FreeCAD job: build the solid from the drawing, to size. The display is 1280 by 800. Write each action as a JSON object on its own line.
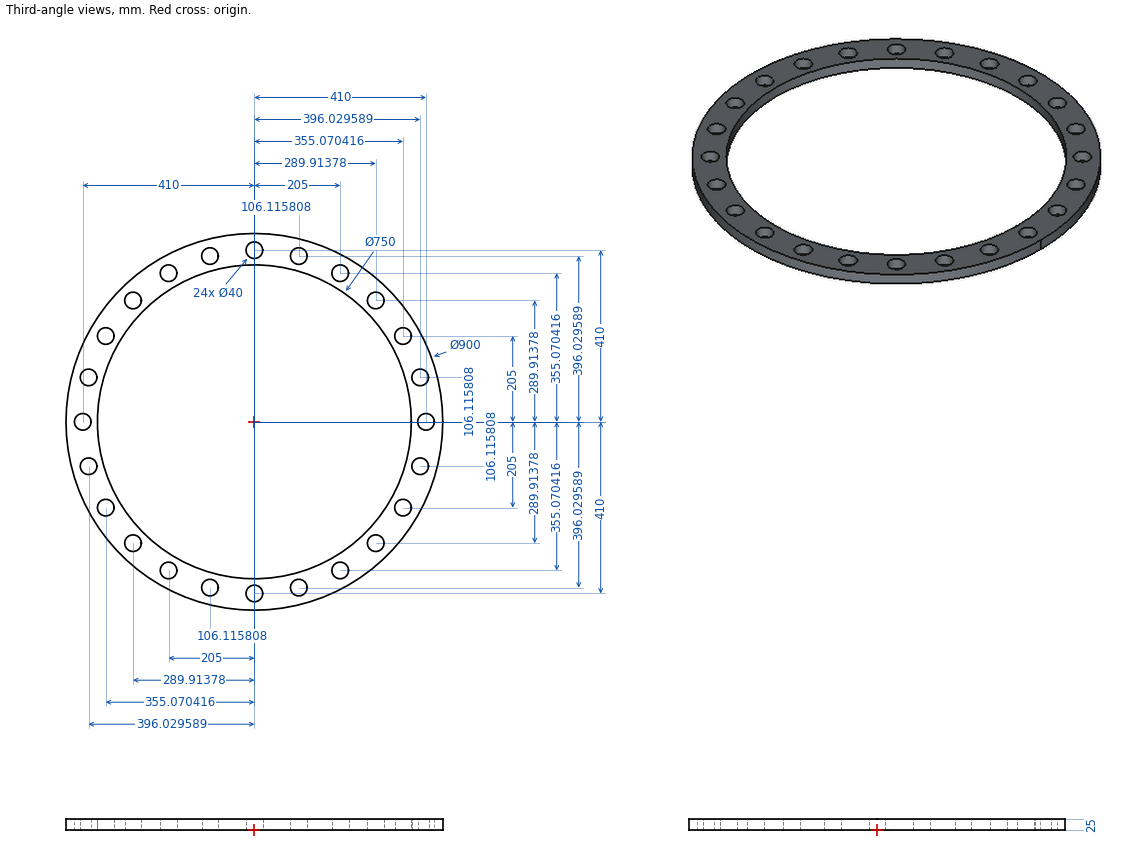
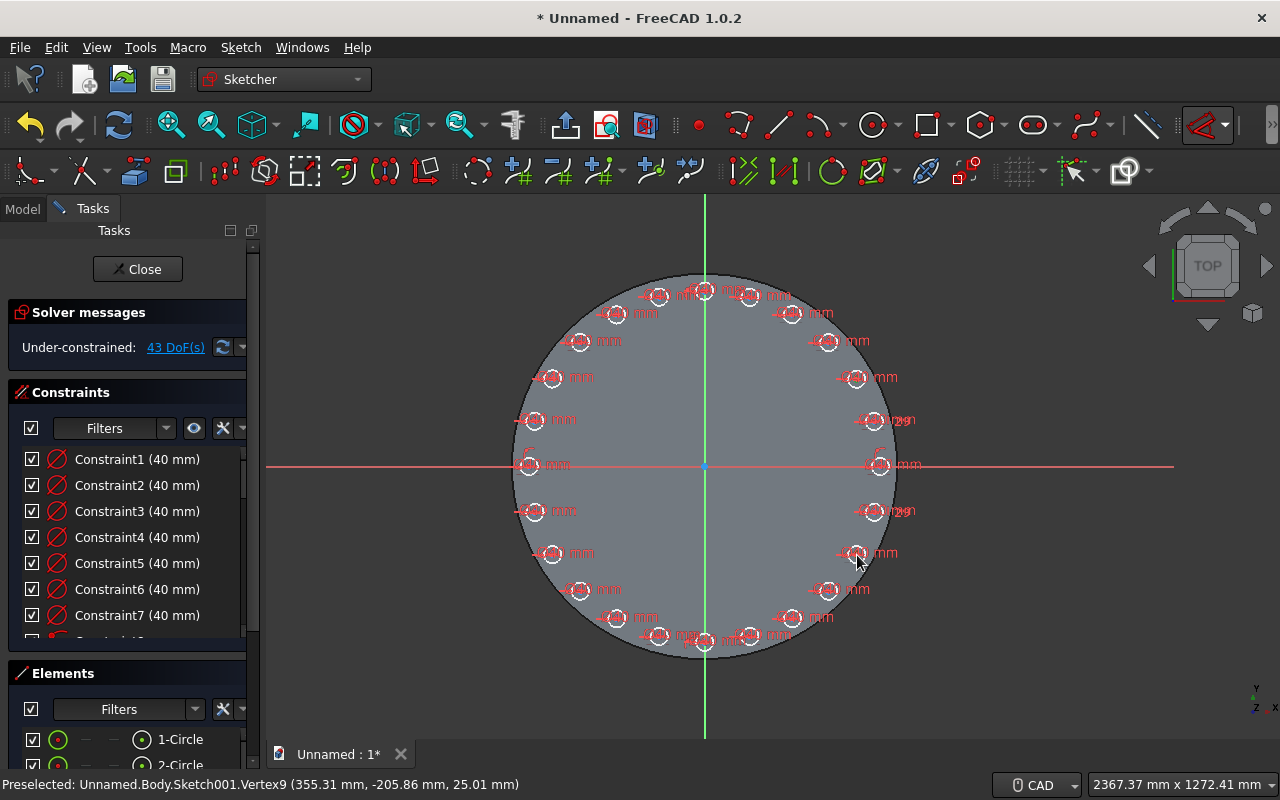
{"action": "key", "text": "v"}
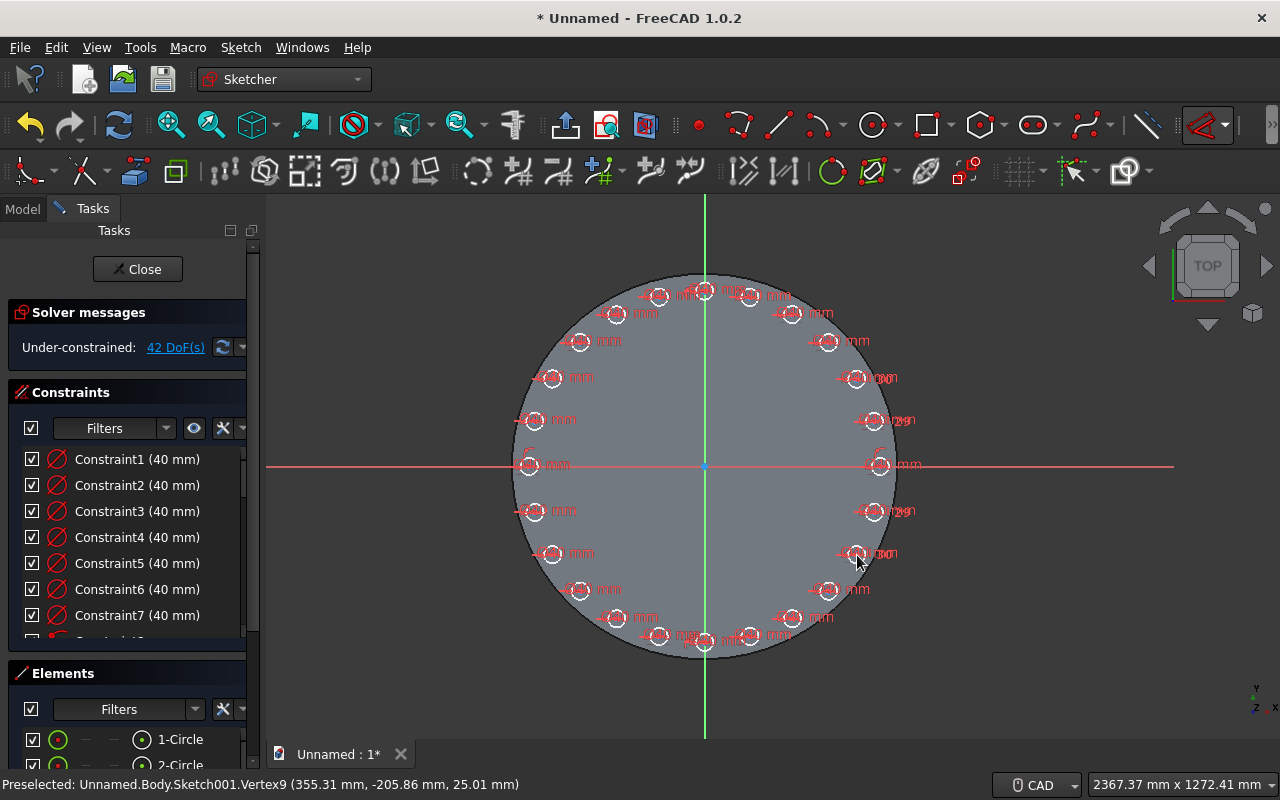
{"action": "left_click", "coordinate": [829, 343]}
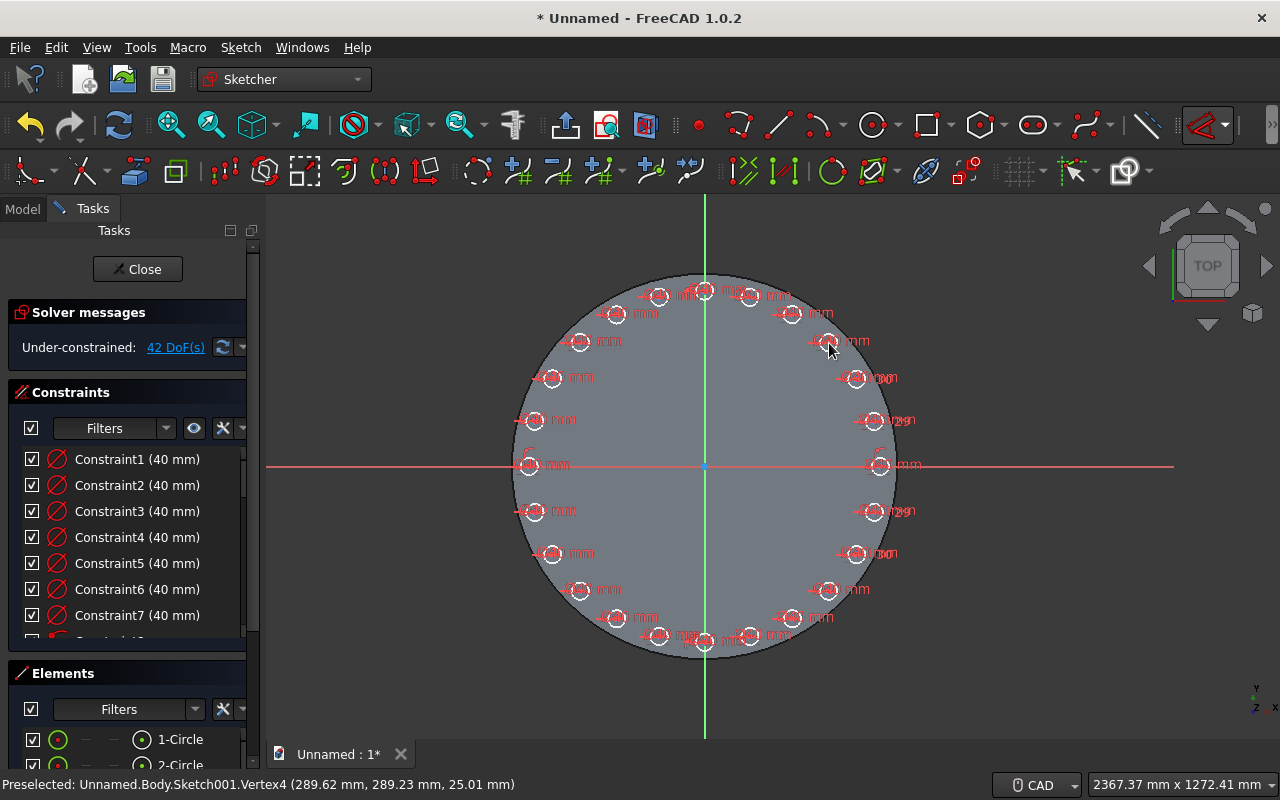
{"action": "left_click", "coordinate": [829, 591]}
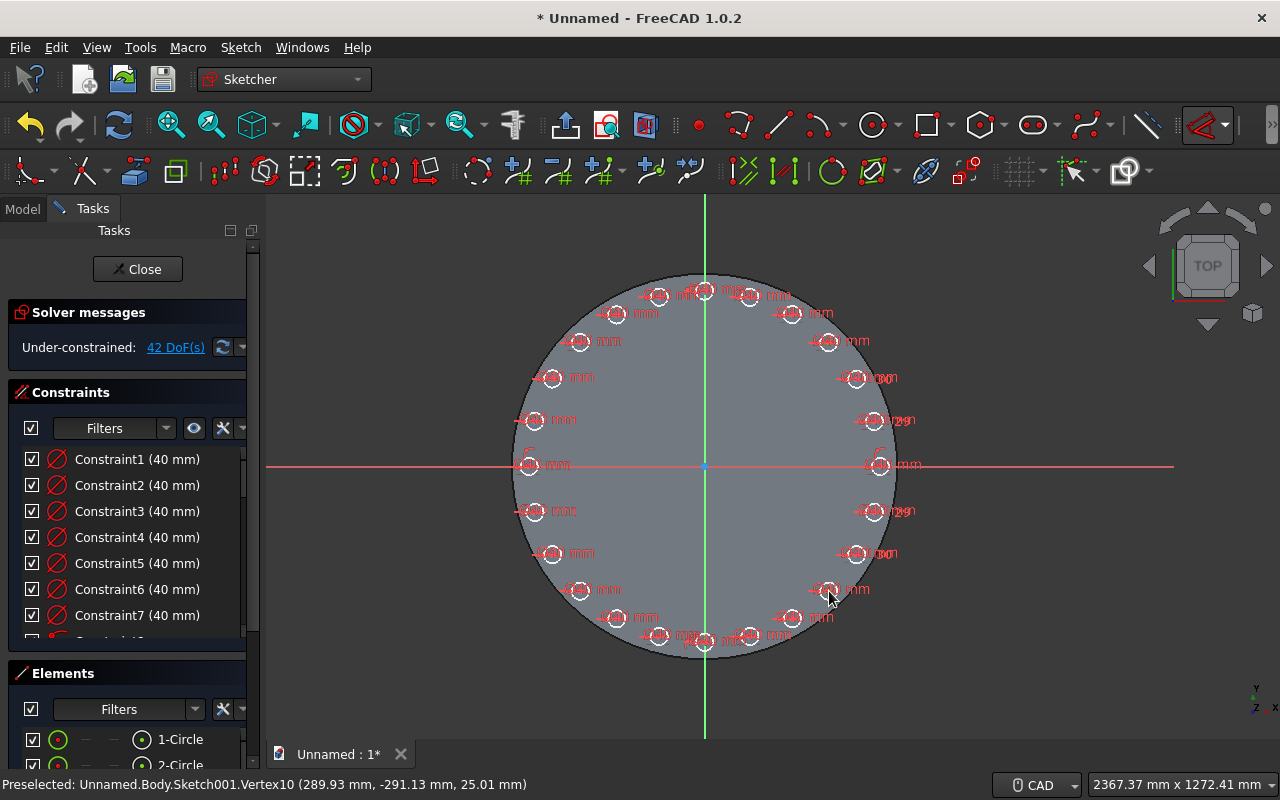
{"action": "key", "text": "v"}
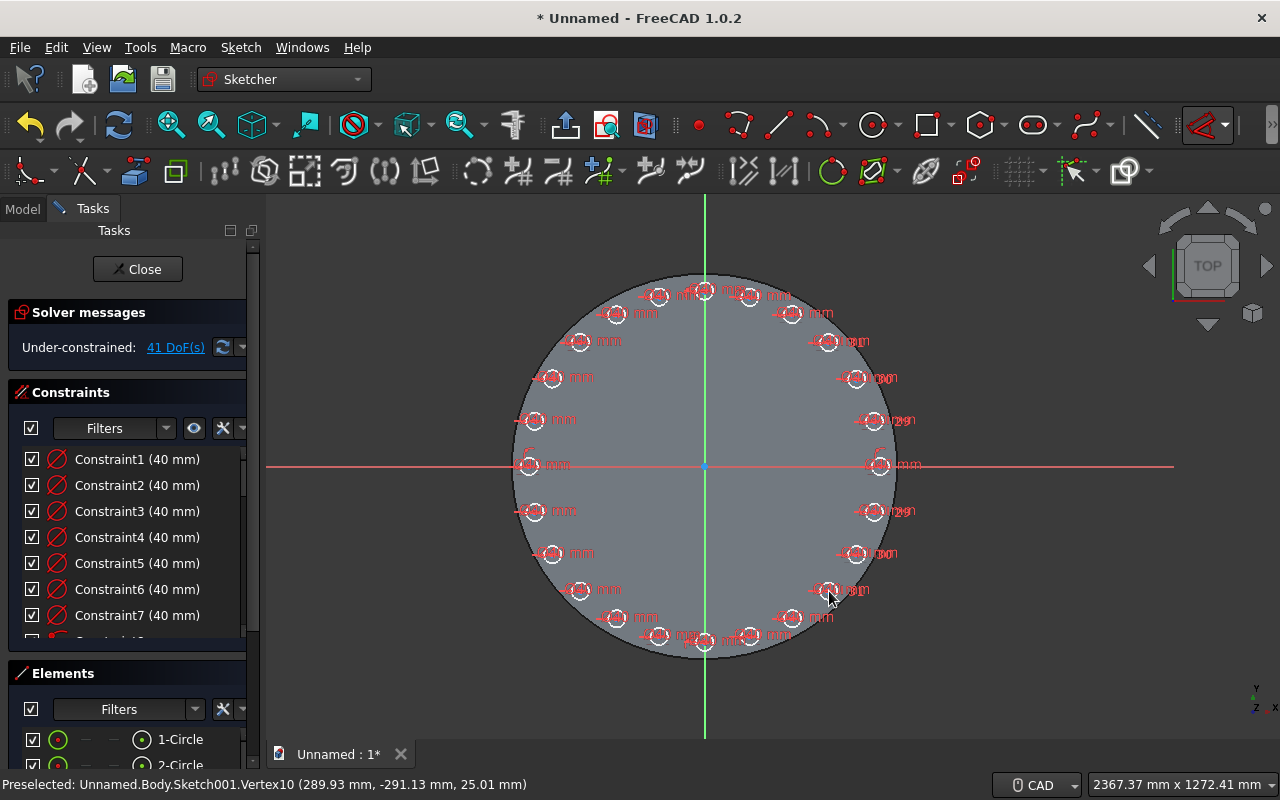
{"action": "left_click", "coordinate": [750, 637]}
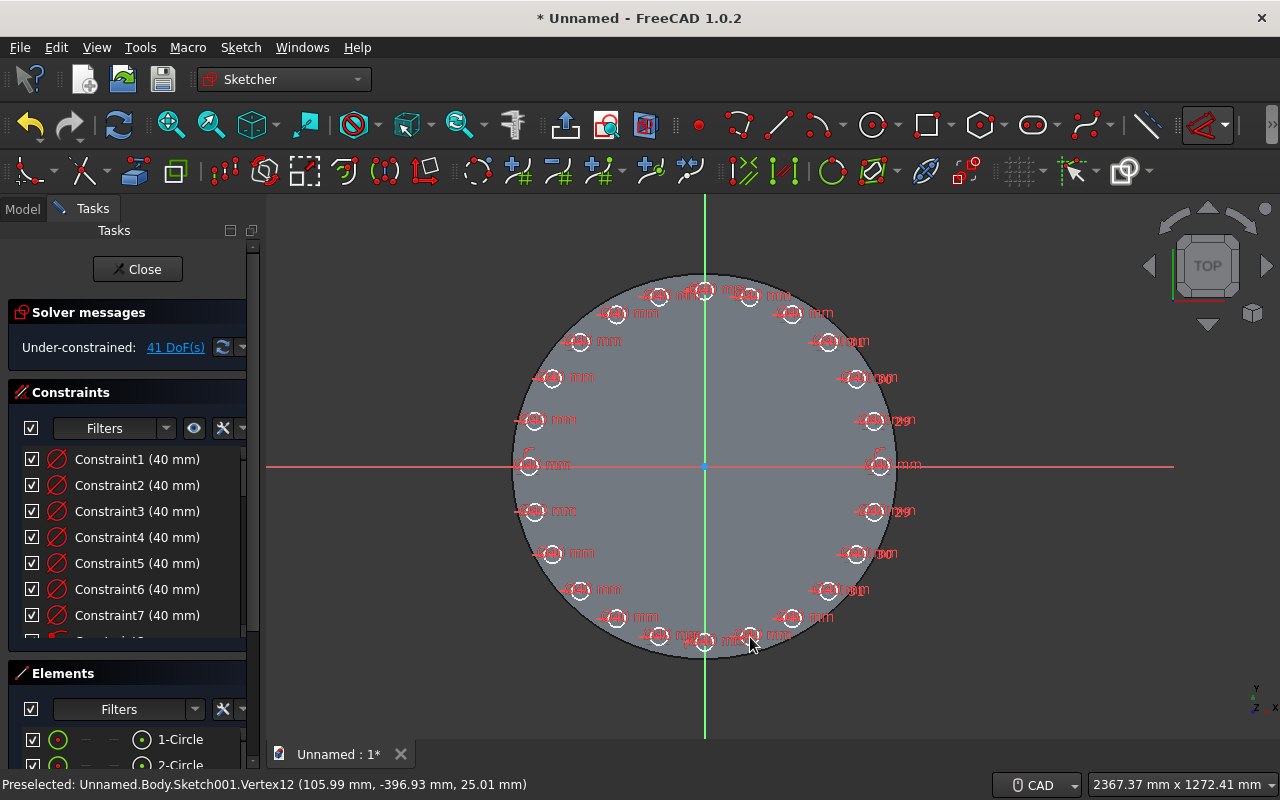
{"action": "left_click", "coordinate": [659, 637]}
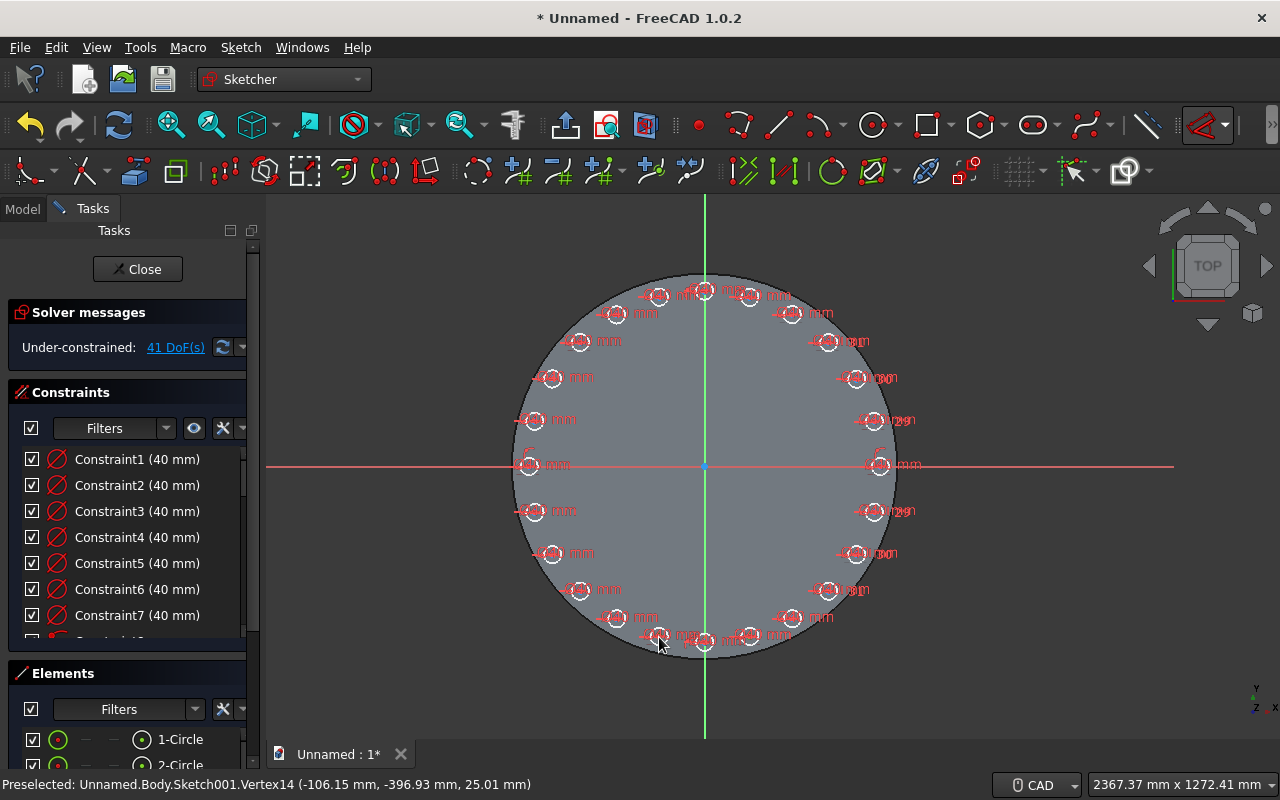
{"action": "key", "text": "h"}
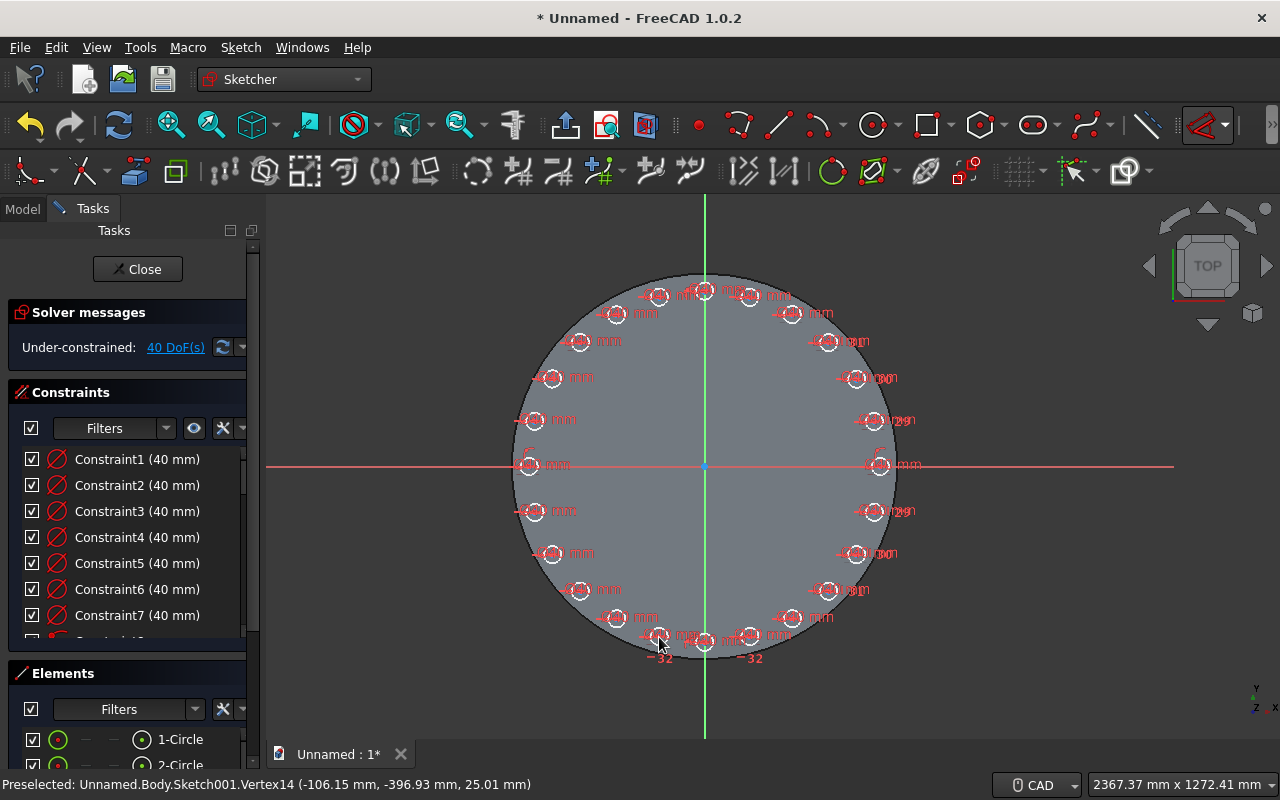
{"action": "left_click", "coordinate": [792, 619]}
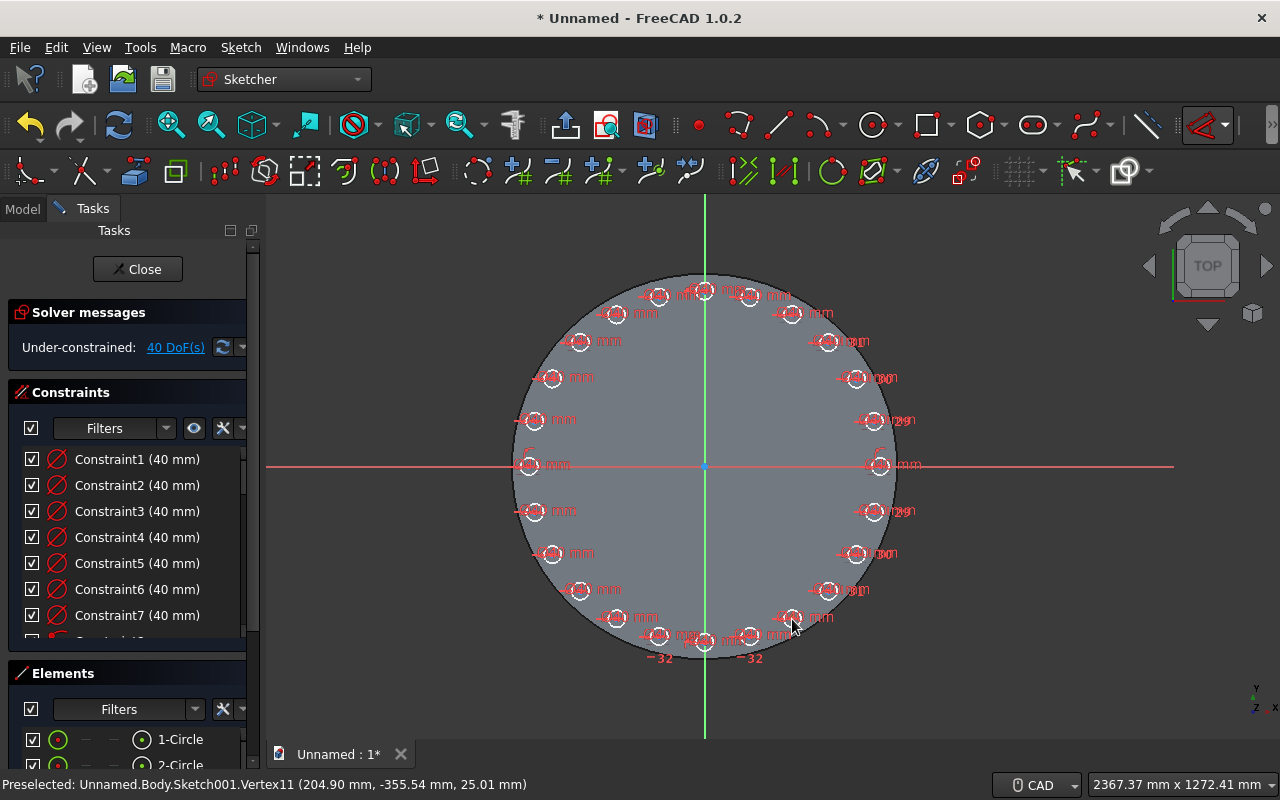
{"action": "left_click", "coordinate": [617, 619]}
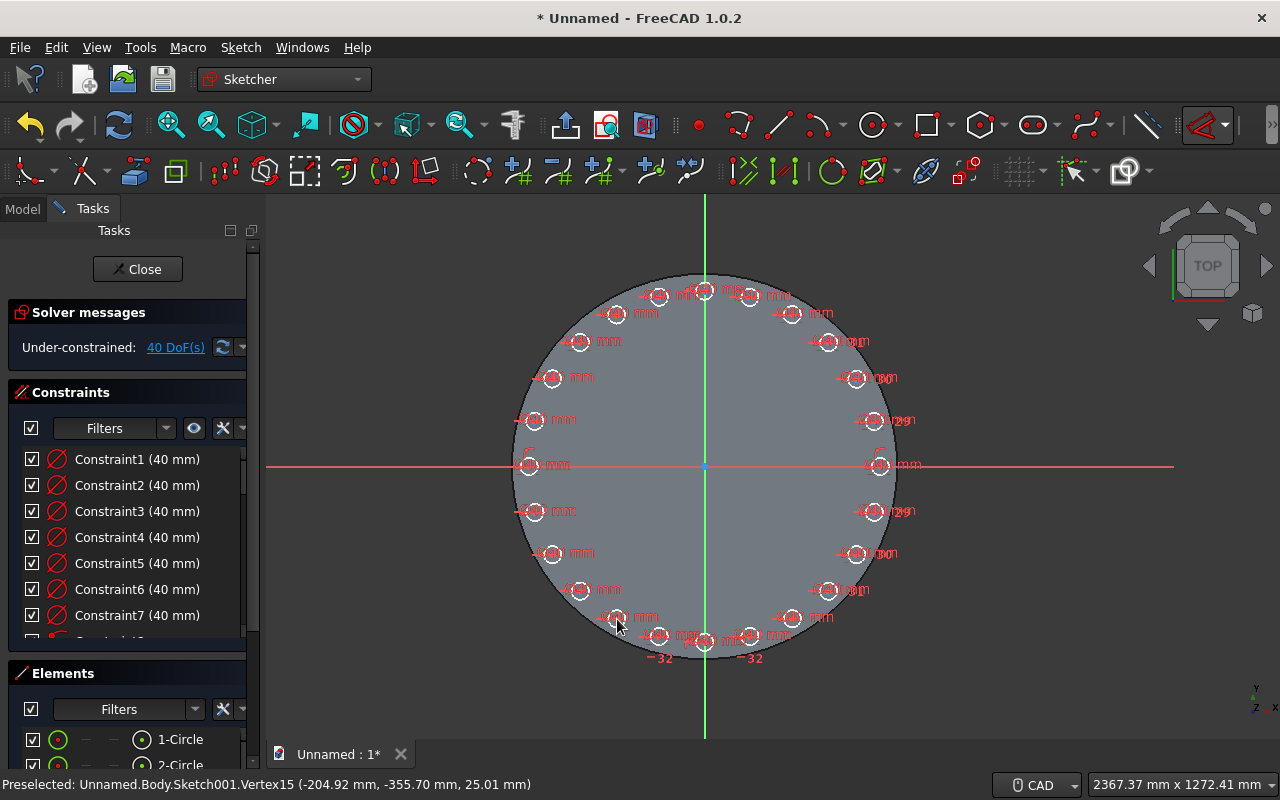
{"action": "key", "text": "h"}